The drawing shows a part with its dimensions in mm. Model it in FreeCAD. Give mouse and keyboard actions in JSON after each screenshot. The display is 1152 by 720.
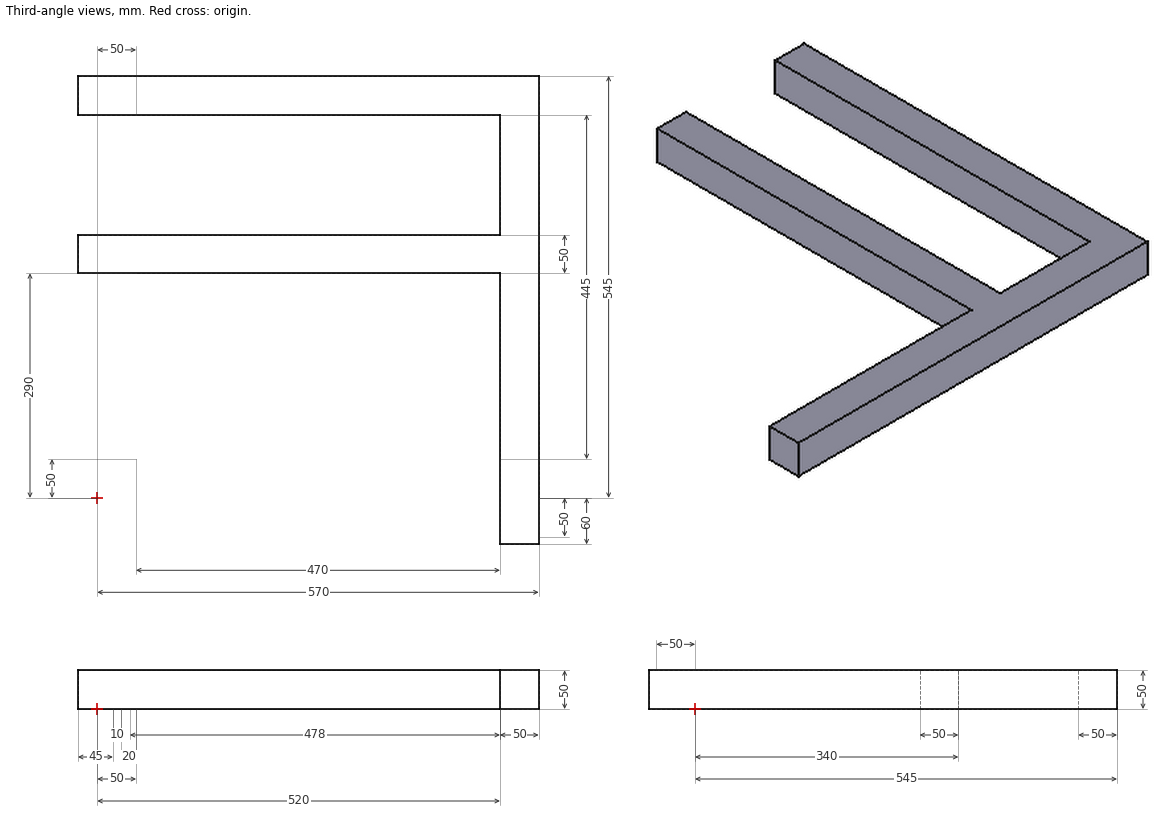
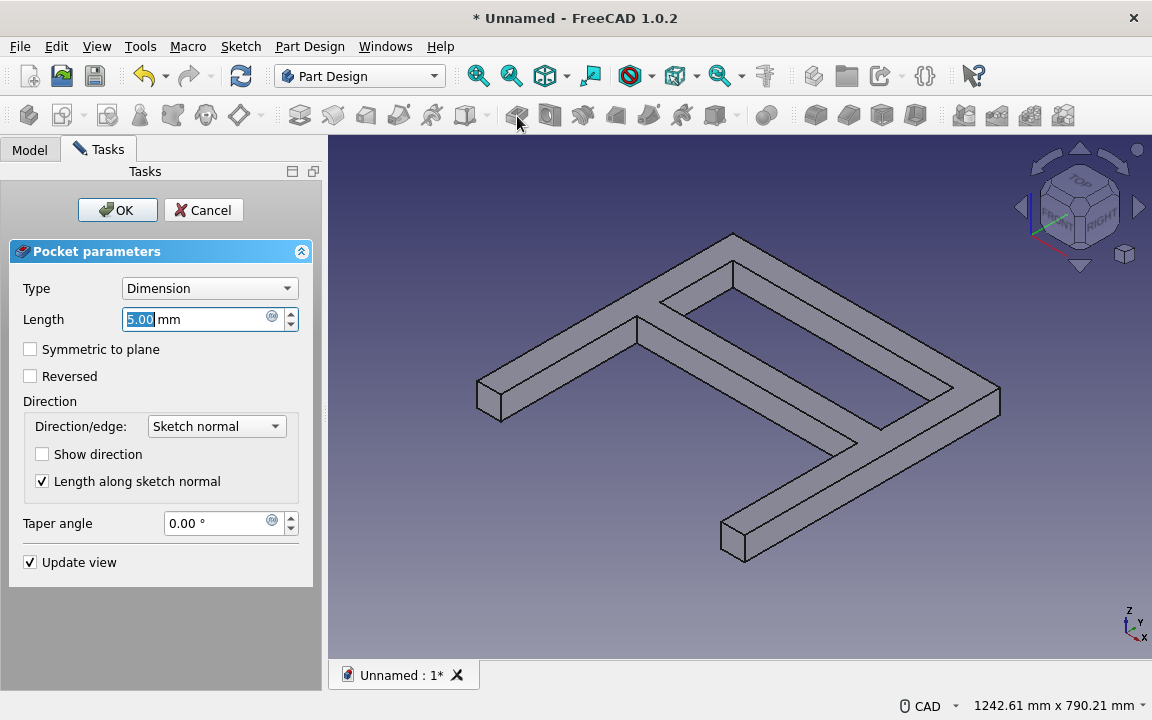
{"action": "type", "text": "50"}
{"action": "key", "text": "Tab"}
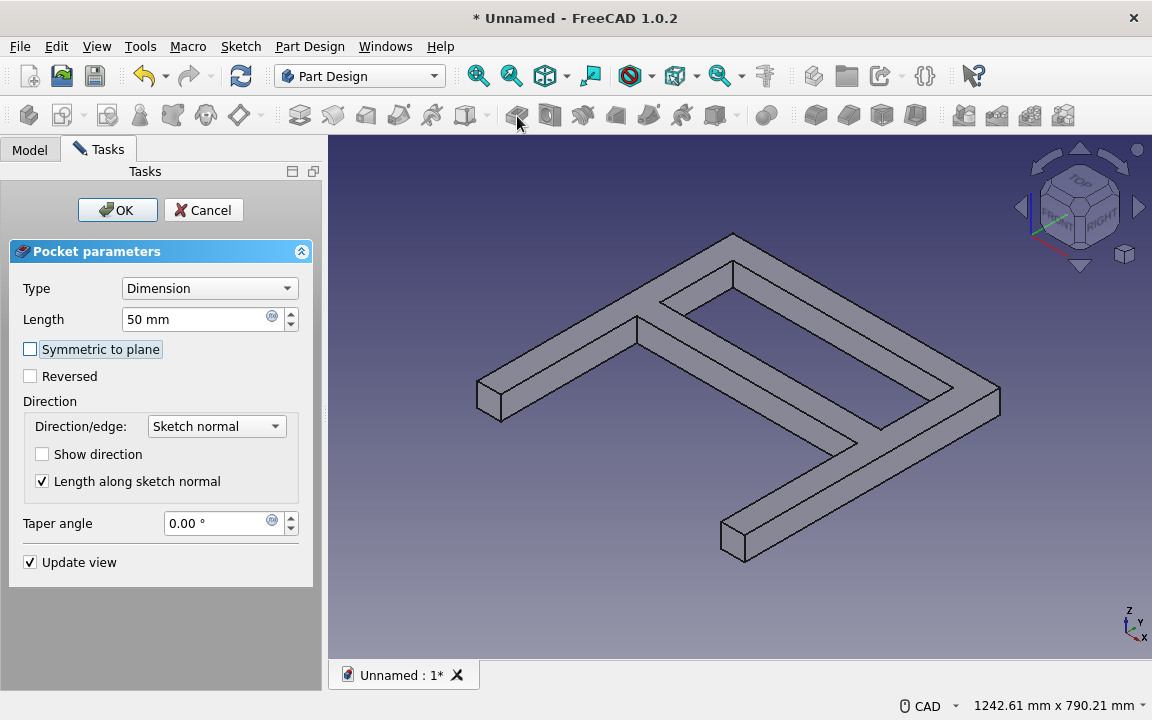
{"action": "left_click", "coordinate": [31, 376]}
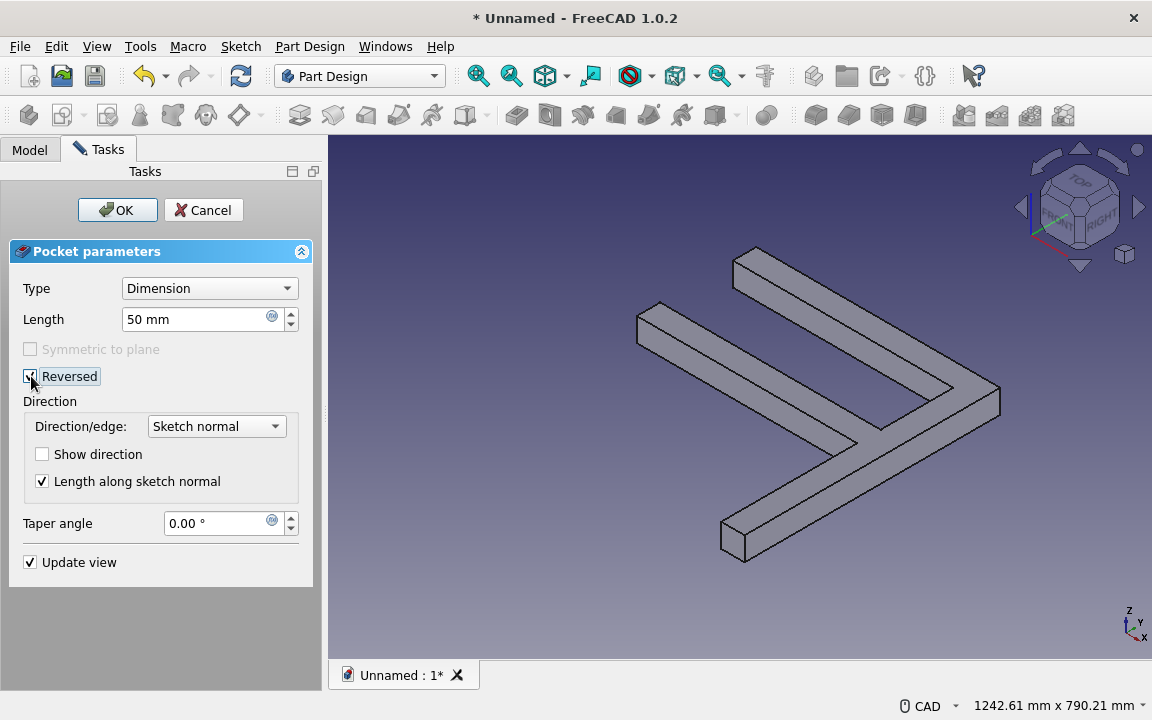
{"action": "left_click", "coordinate": [118, 210]}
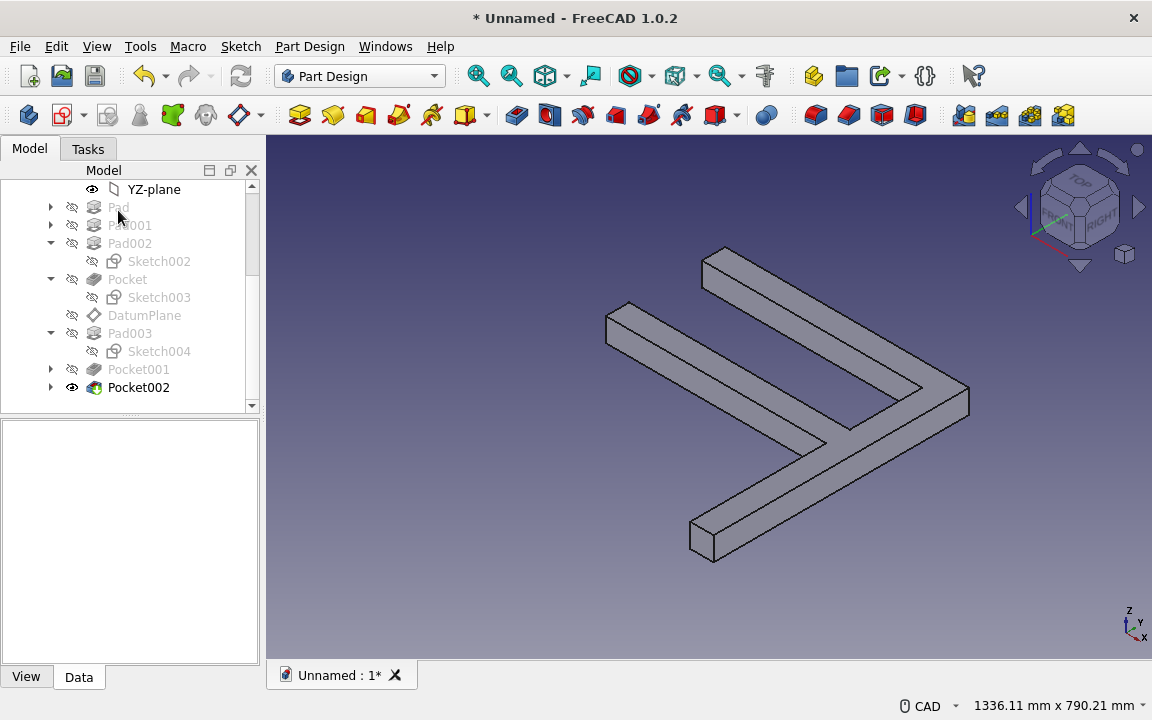
{"action": "key", "text": "6"}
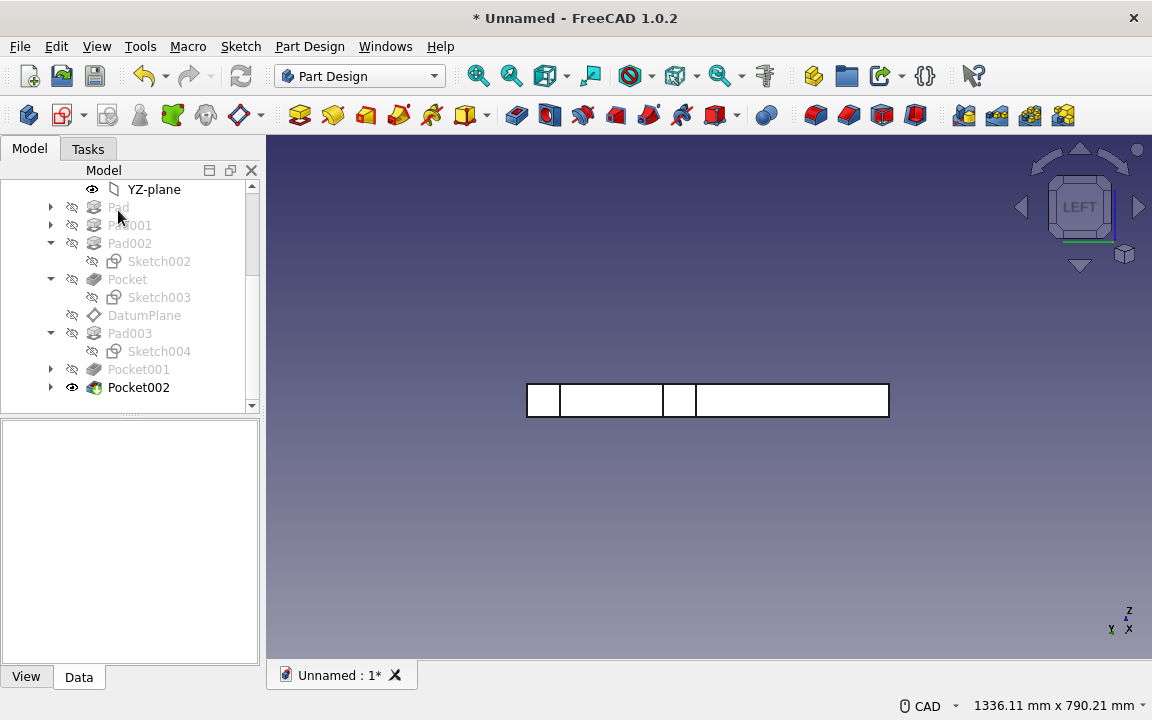
{"action": "left_click", "coordinate": [479, 76]}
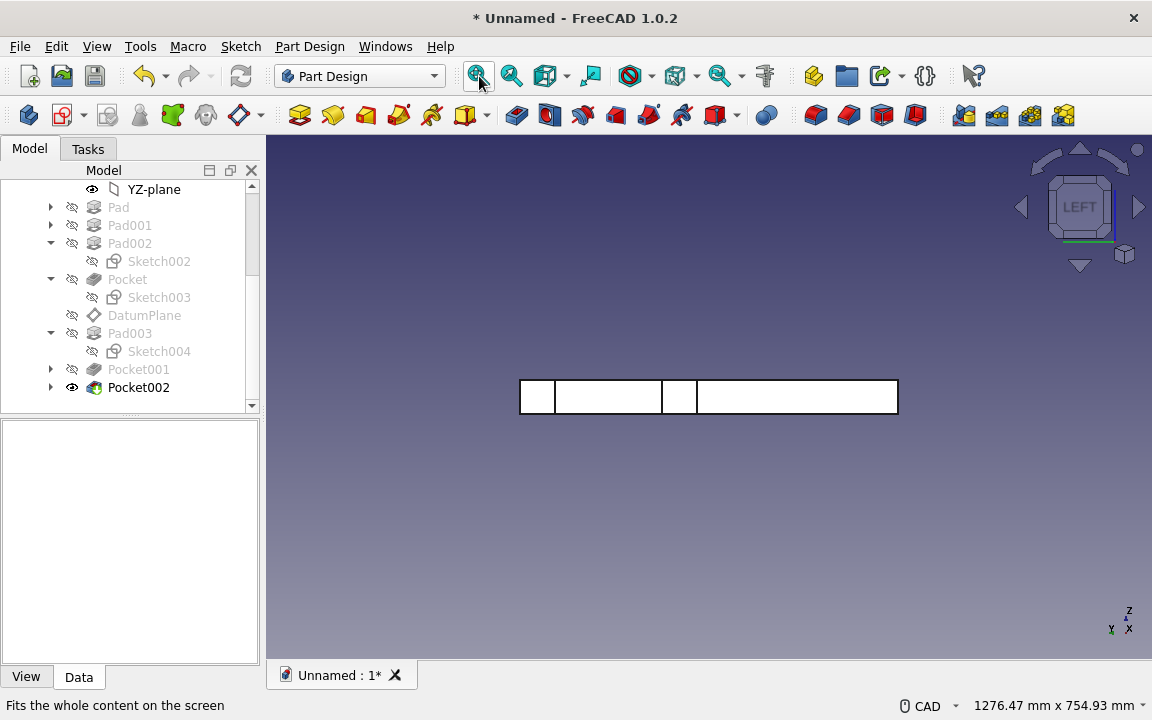
{"action": "left_click", "coordinate": [537, 396]}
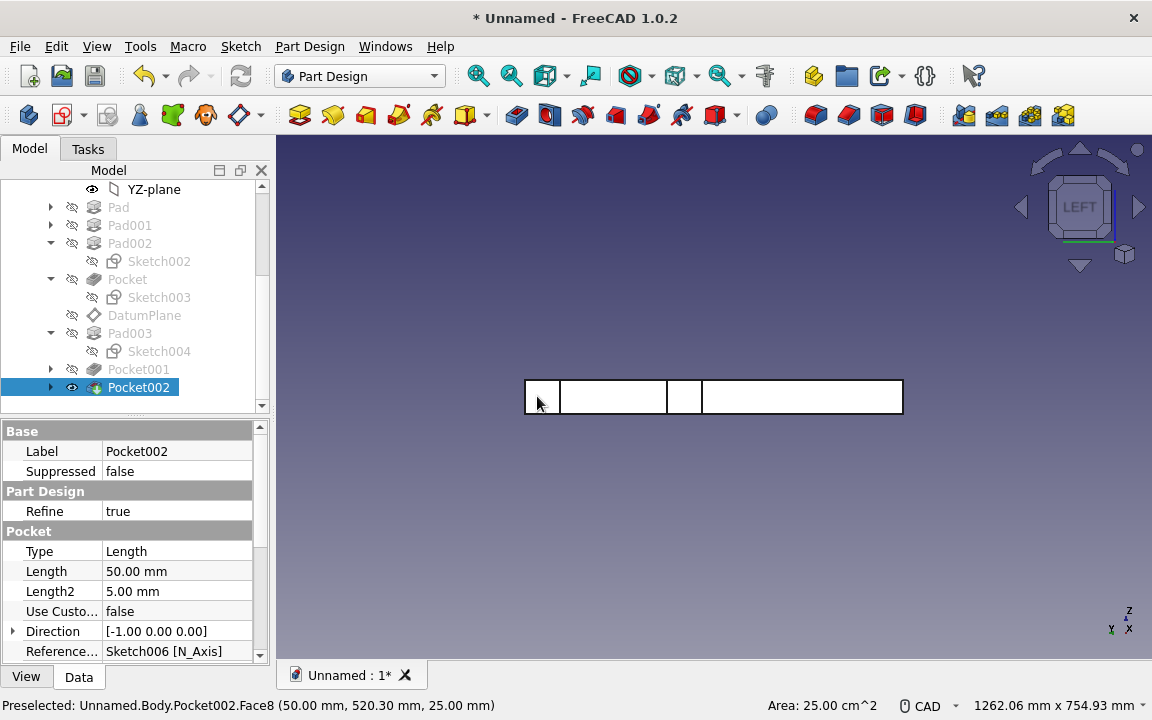
{"action": "left_click", "coordinate": [62, 116]}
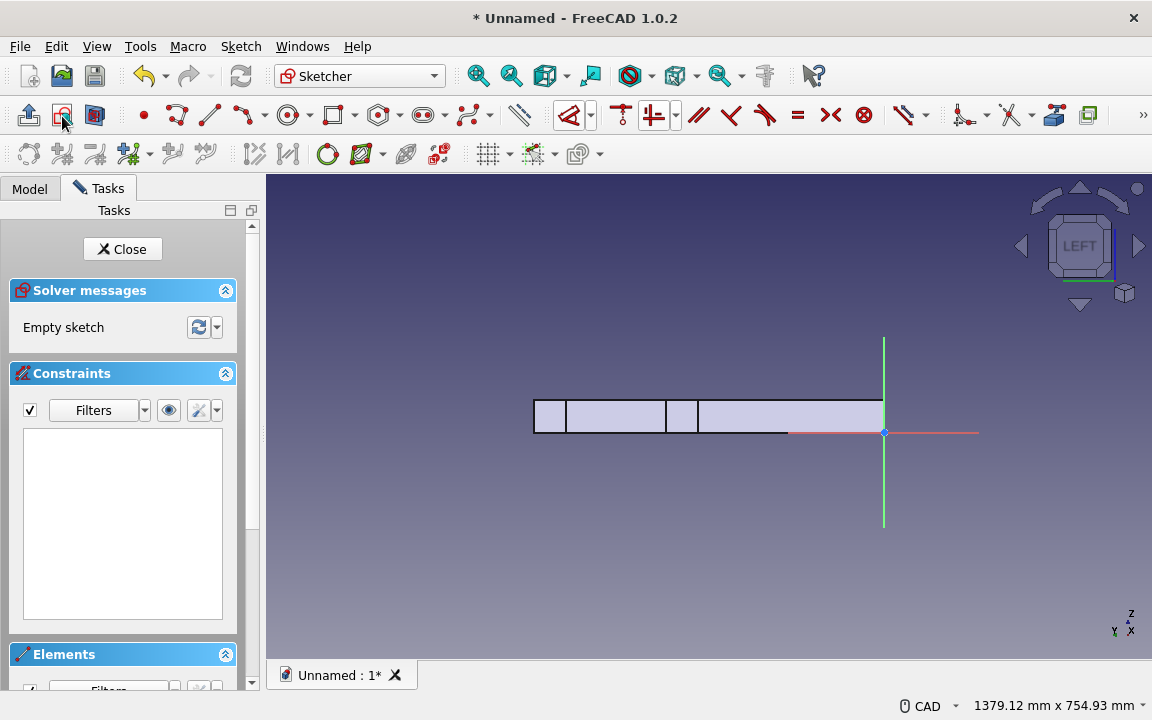
{"action": "scroll", "coordinate": [848, 416], "scroll_direction": "up", "scroll_amount": 2}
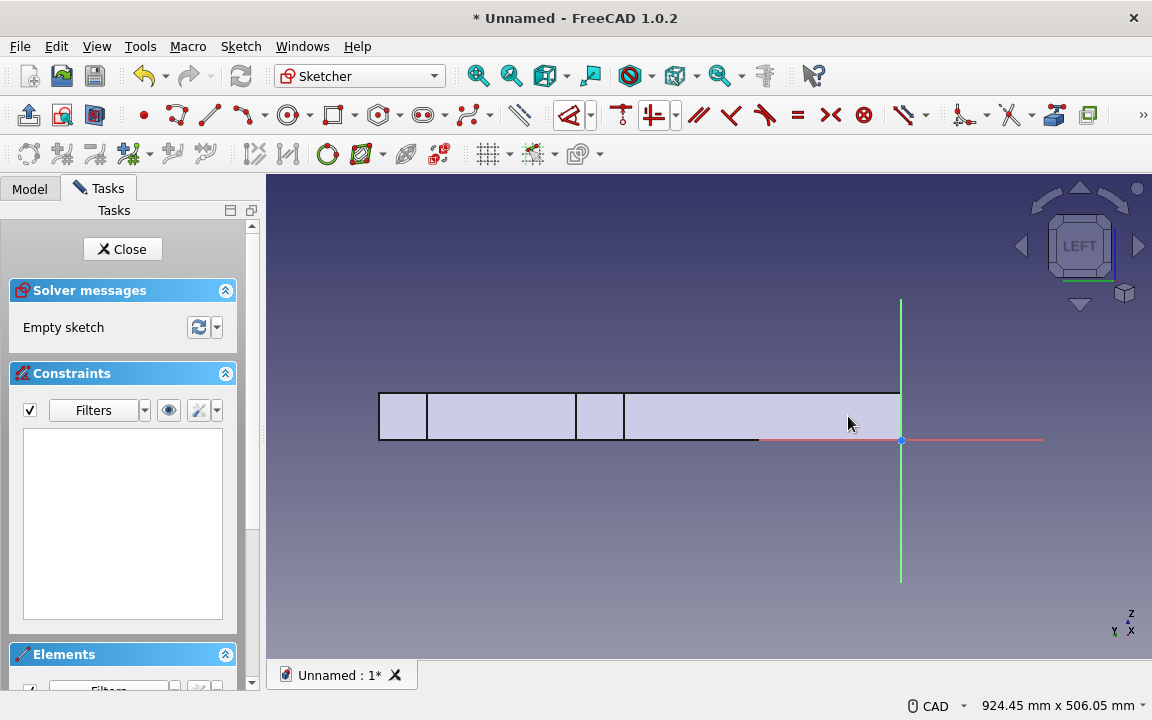
{"action": "key", "text": "g r"}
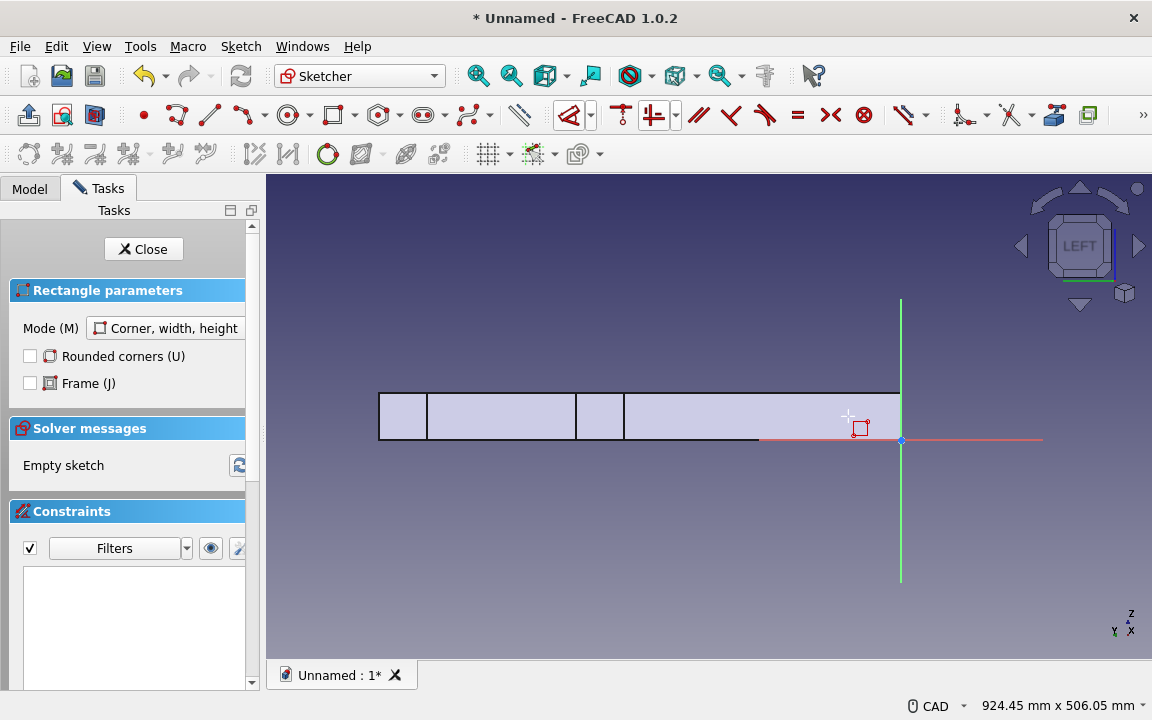
{"action": "left_click", "coordinate": [379, 393]}
{"action": "left_click", "coordinate": [427, 440]}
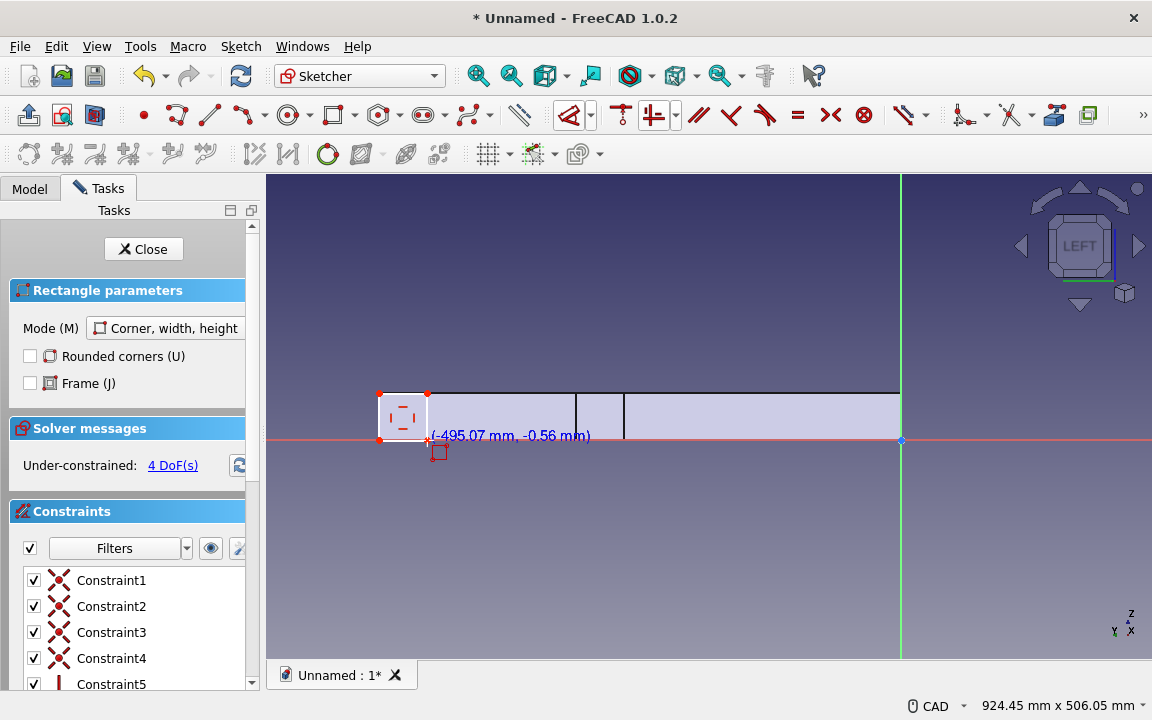
{"action": "left_click", "coordinate": [576, 393]}
{"action": "left_click", "coordinate": [624, 440]}
{"action": "key", "text": "Escape"}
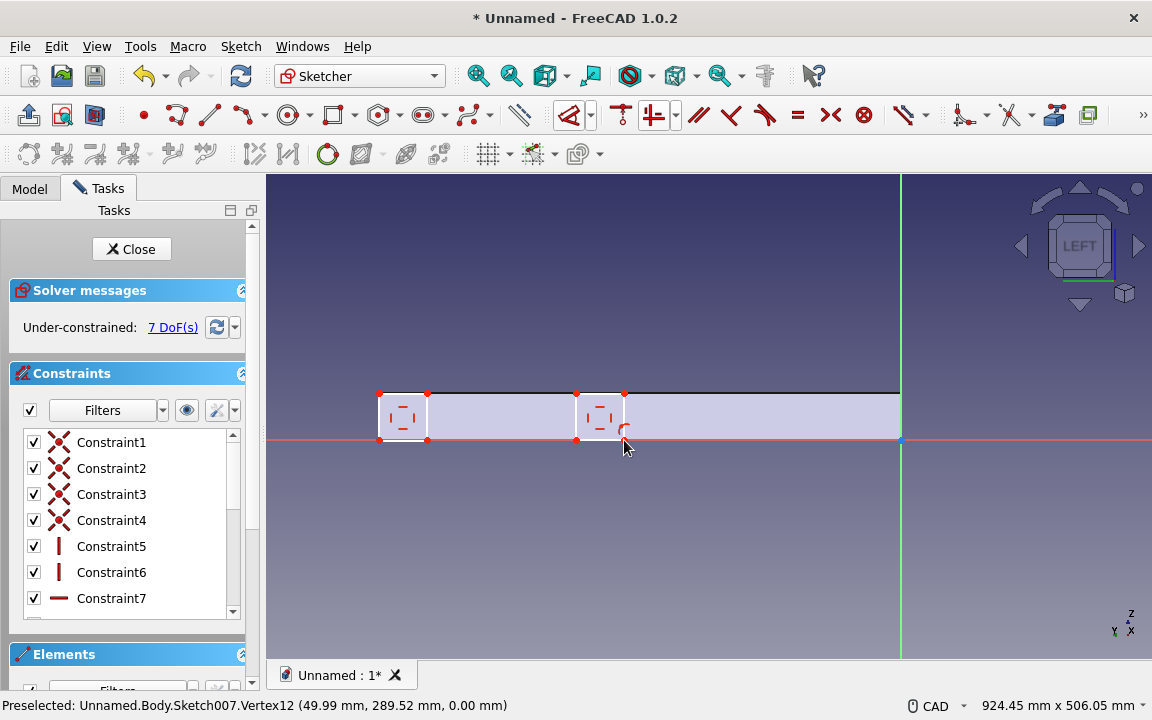
{"action": "left_click", "coordinate": [379, 441]}